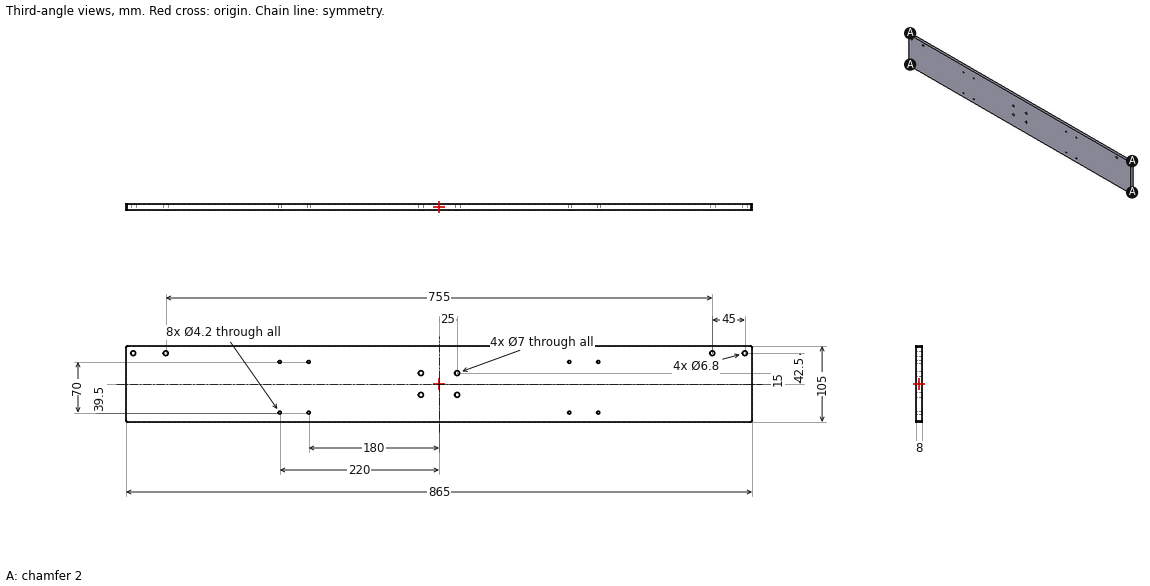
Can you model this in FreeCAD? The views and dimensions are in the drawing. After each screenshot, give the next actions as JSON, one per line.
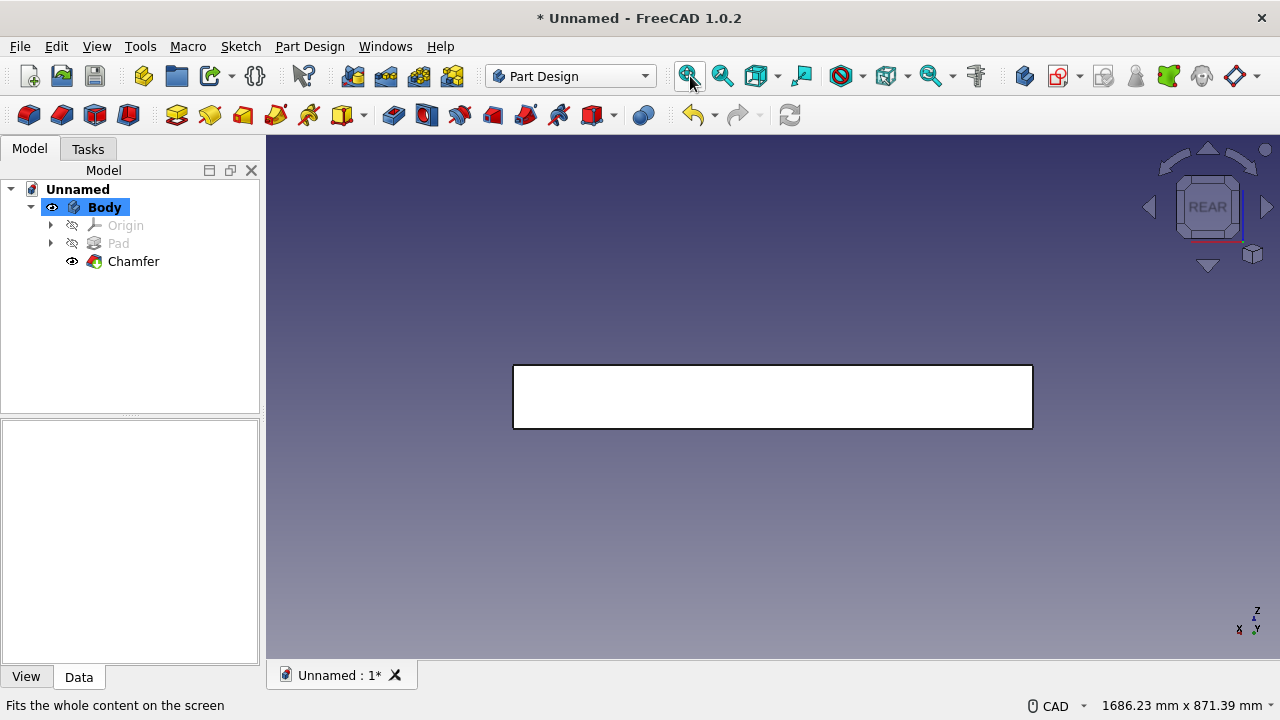
{"action": "left_click", "coordinate": [550, 396]}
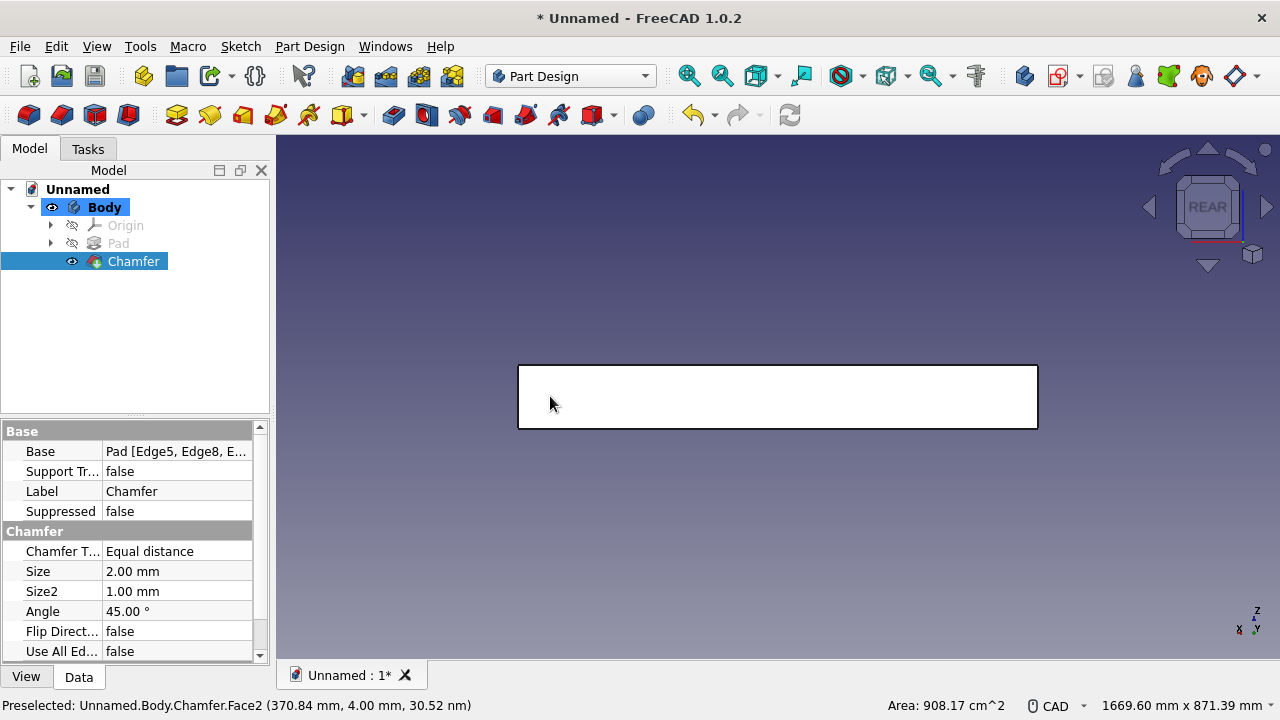
{"action": "left_click", "coordinate": [1058, 76]}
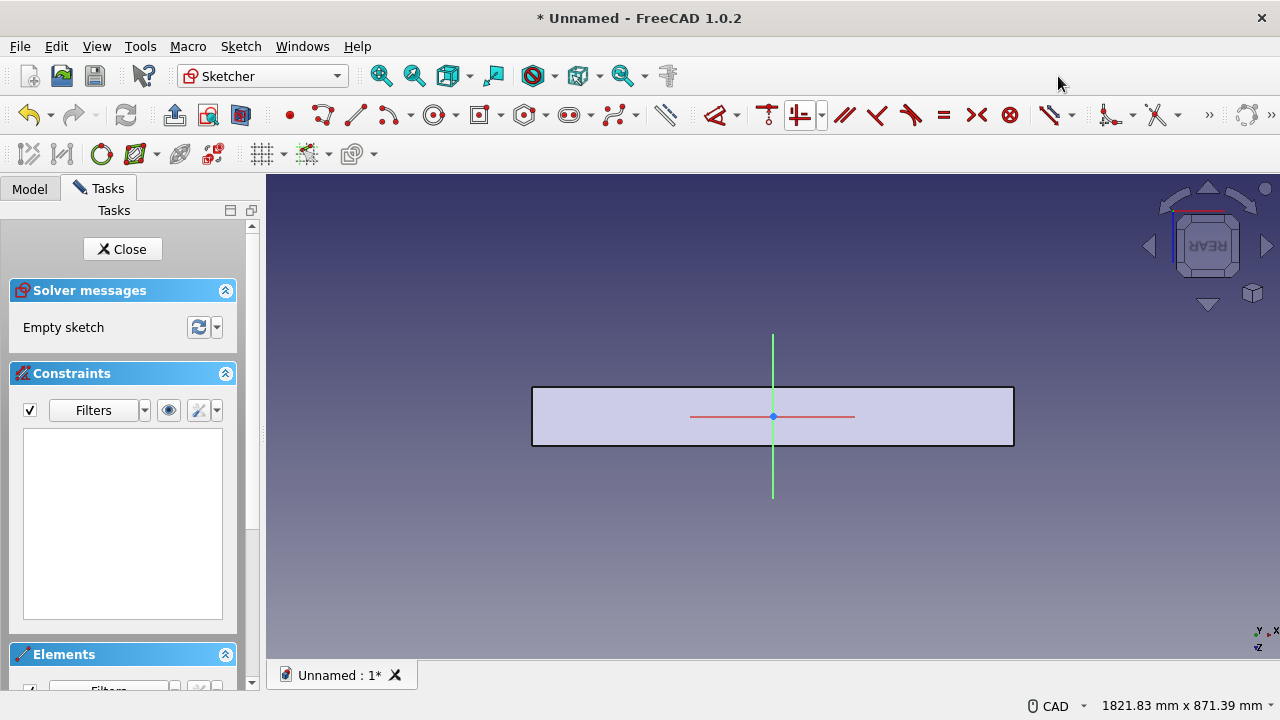
{"action": "scroll", "coordinate": [829, 412], "scroll_direction": "up", "scroll_amount": 4}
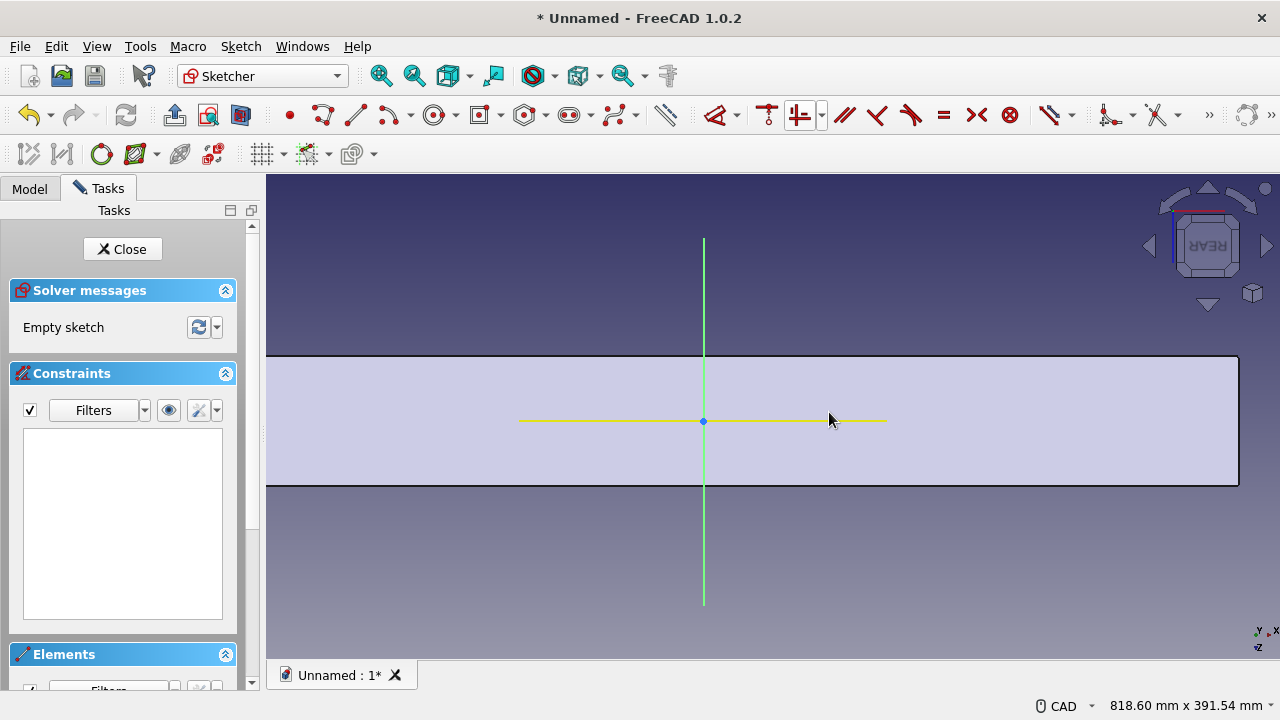
{"action": "left_click", "coordinate": [434, 116]}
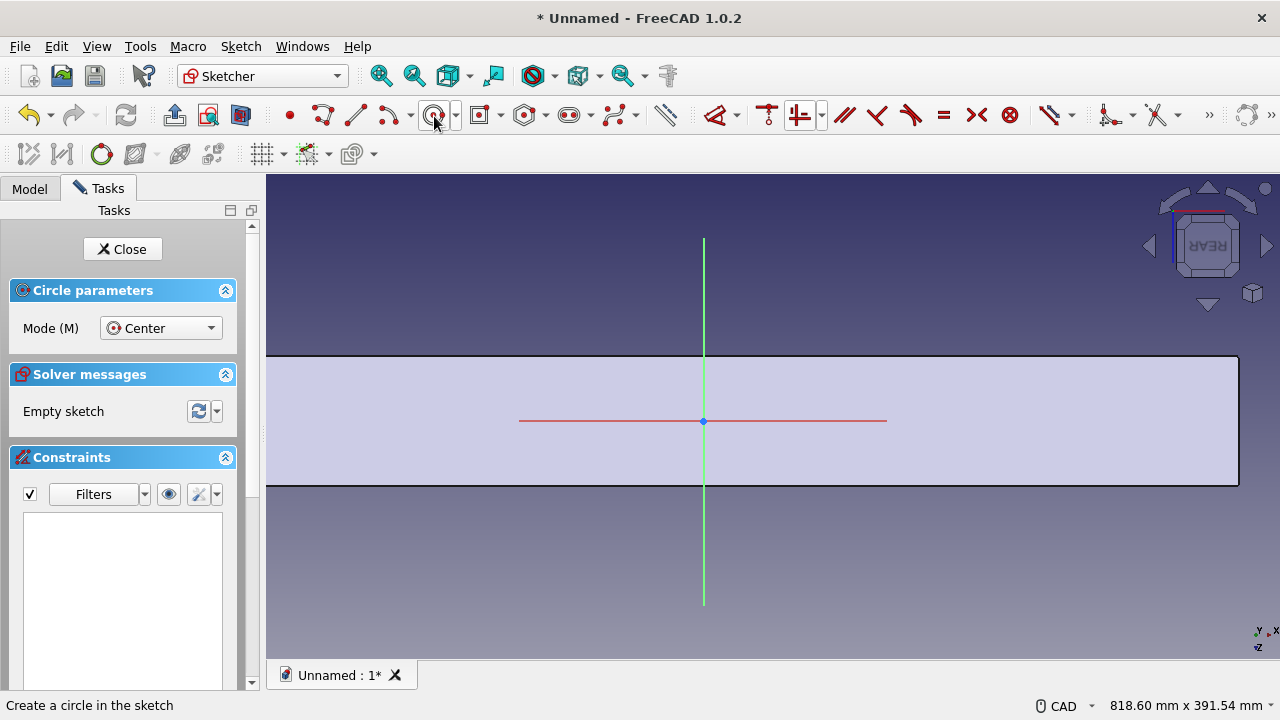
{"action": "scroll", "coordinate": [431, 372], "scroll_direction": "up", "scroll_amount": 11}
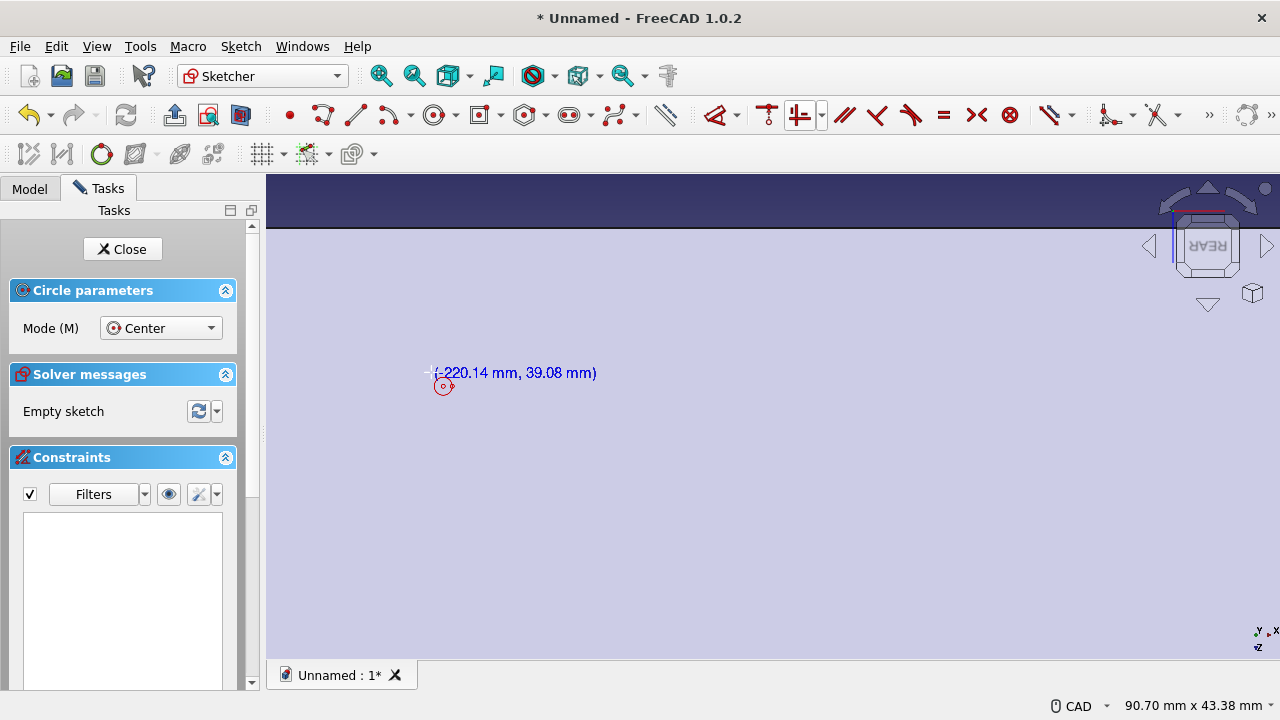
{"action": "scroll", "coordinate": [432, 373], "scroll_direction": "down", "scroll_amount": 11}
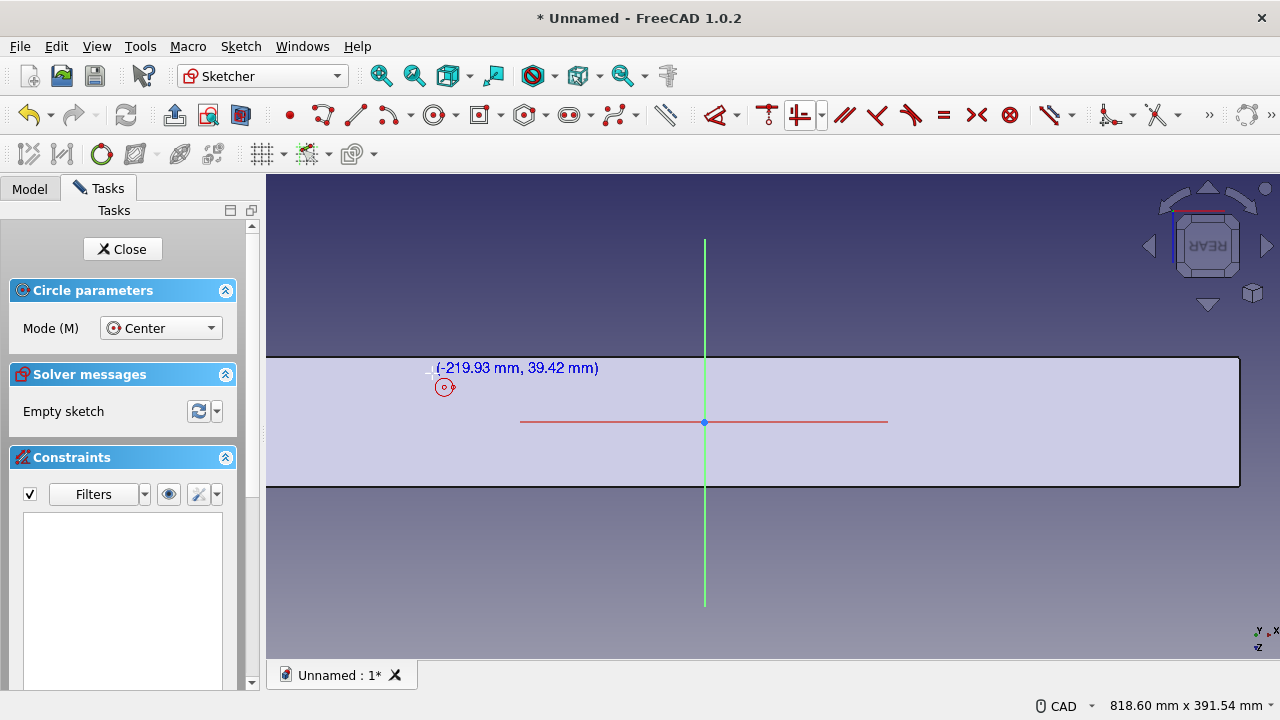
{"action": "left_click", "coordinate": [432, 373]}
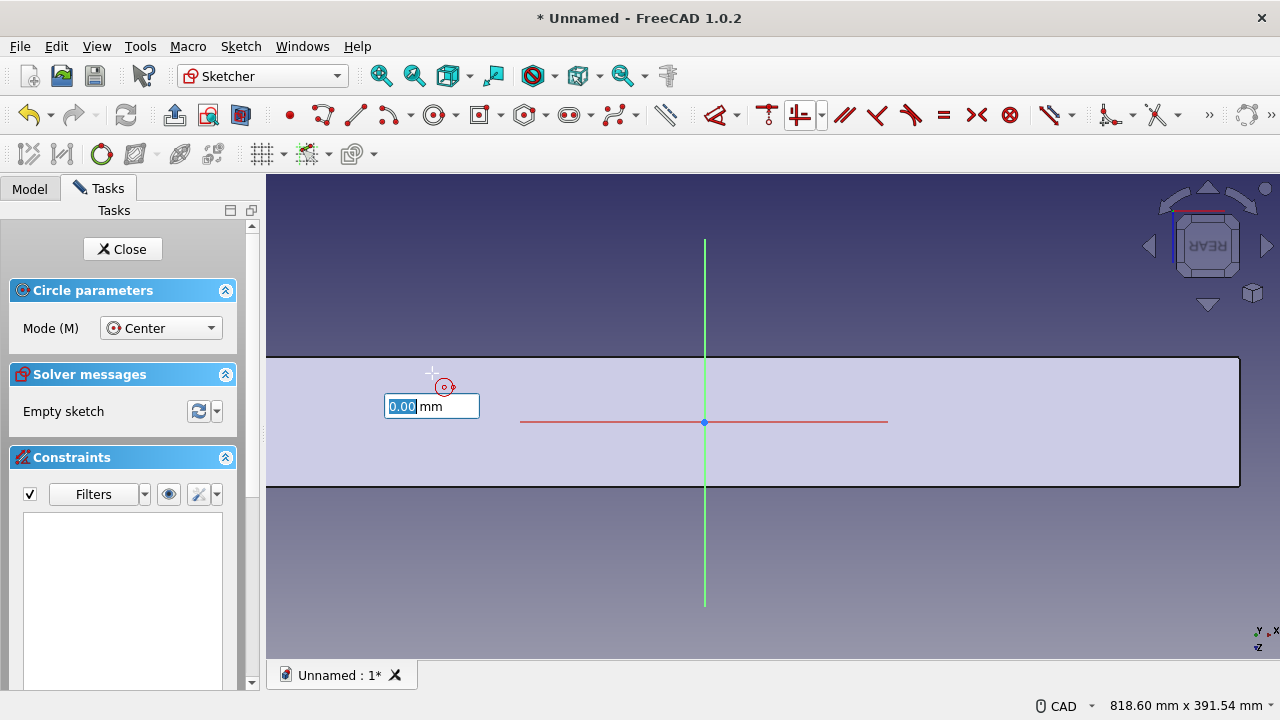
{"action": "scroll", "coordinate": [434, 372], "scroll_direction": "up", "scroll_amount": 10}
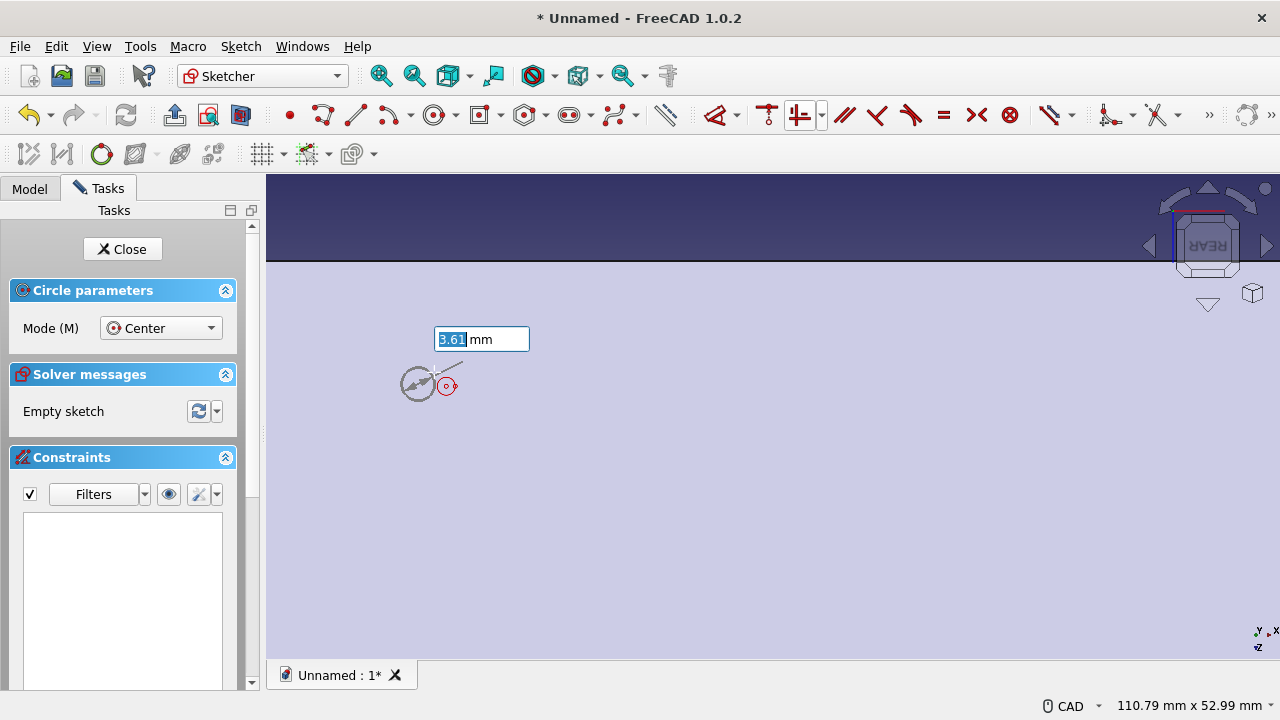
{"action": "left_click", "coordinate": [432, 366]}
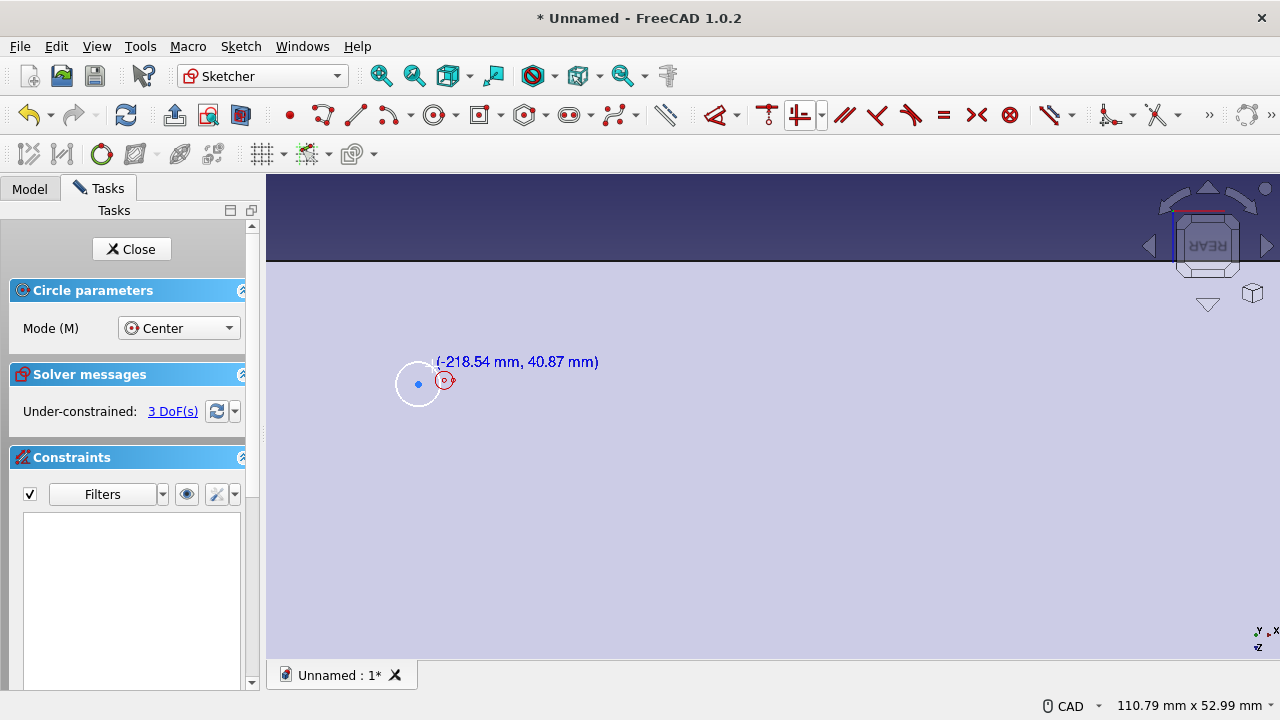
{"action": "scroll", "coordinate": [434, 372], "scroll_direction": "down", "scroll_amount": 10}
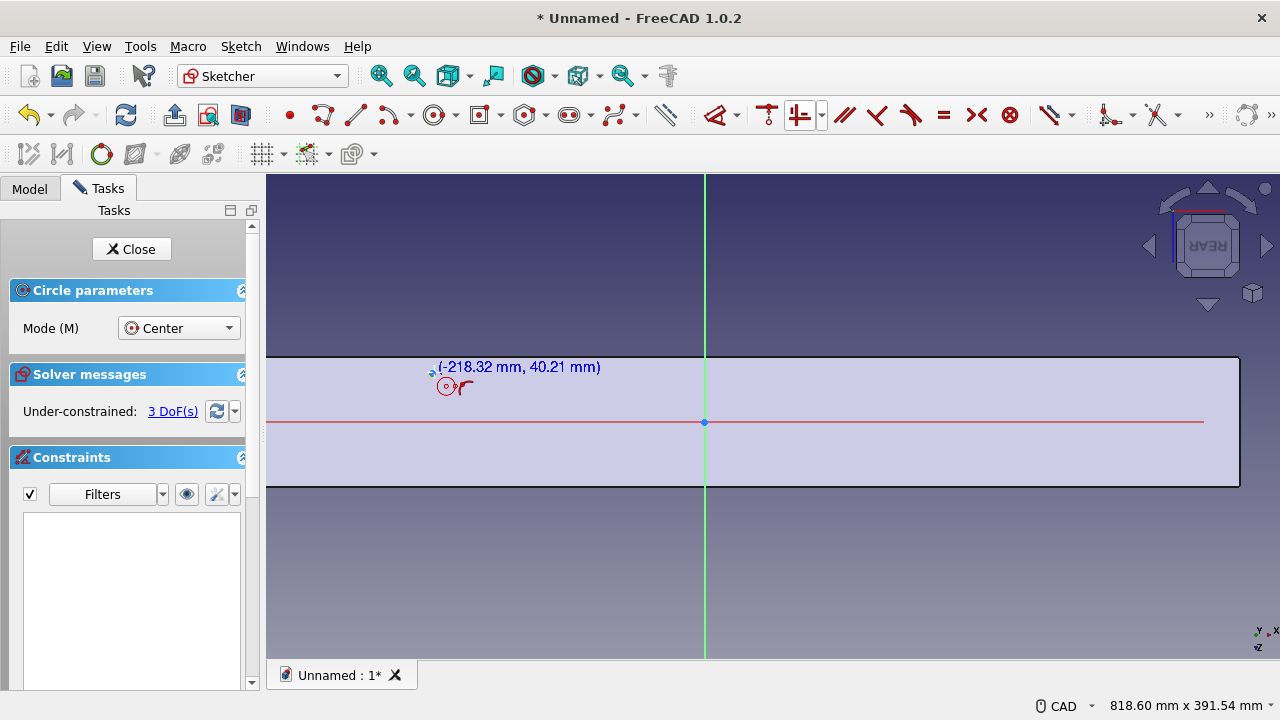
{"action": "left_click", "coordinate": [482, 373]}